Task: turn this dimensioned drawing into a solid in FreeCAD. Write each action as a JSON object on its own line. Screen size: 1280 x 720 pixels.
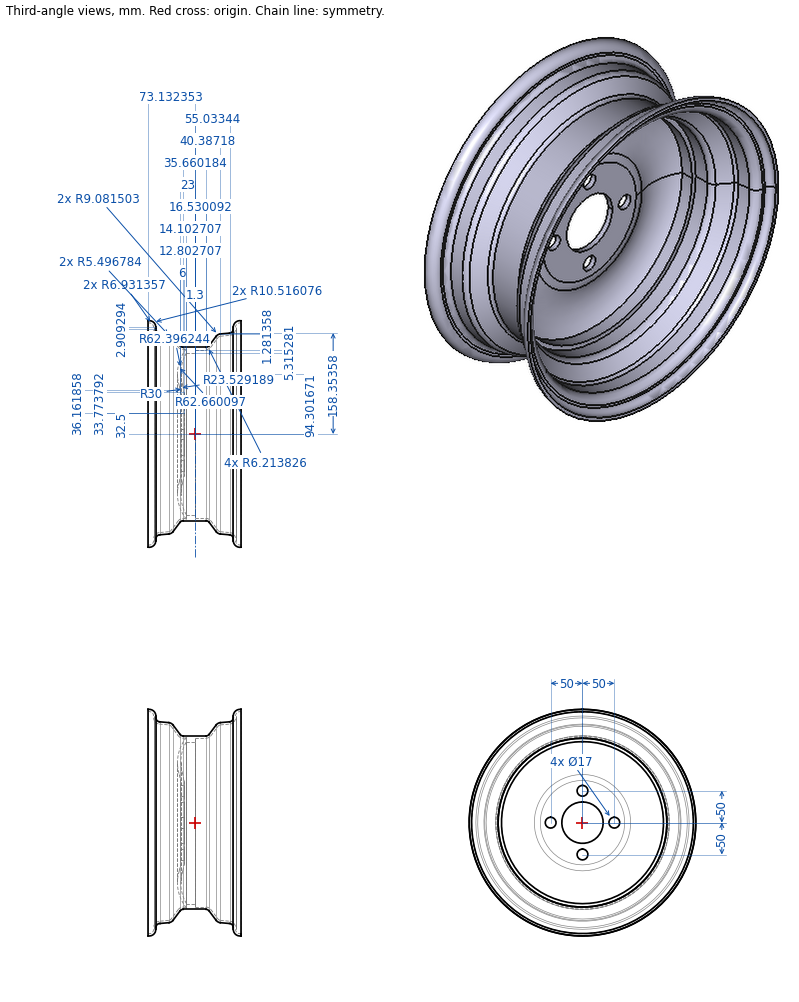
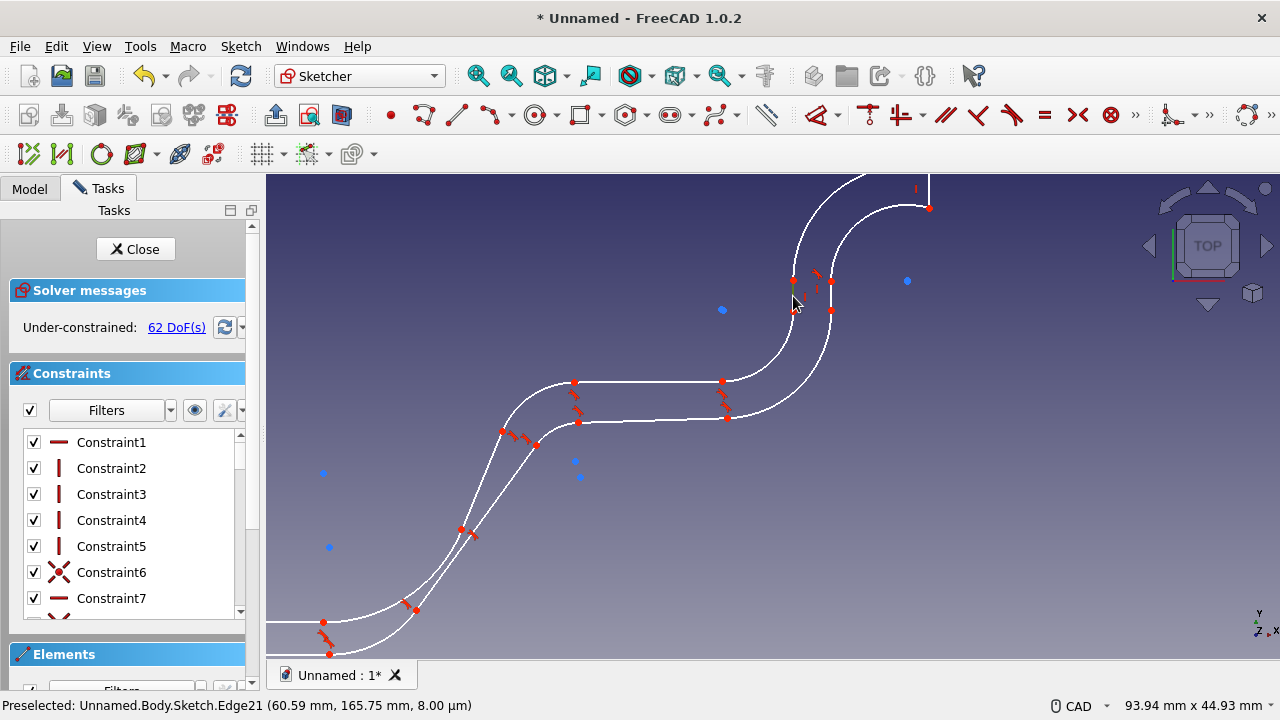
{"action": "left_click", "coordinate": [809, 223]}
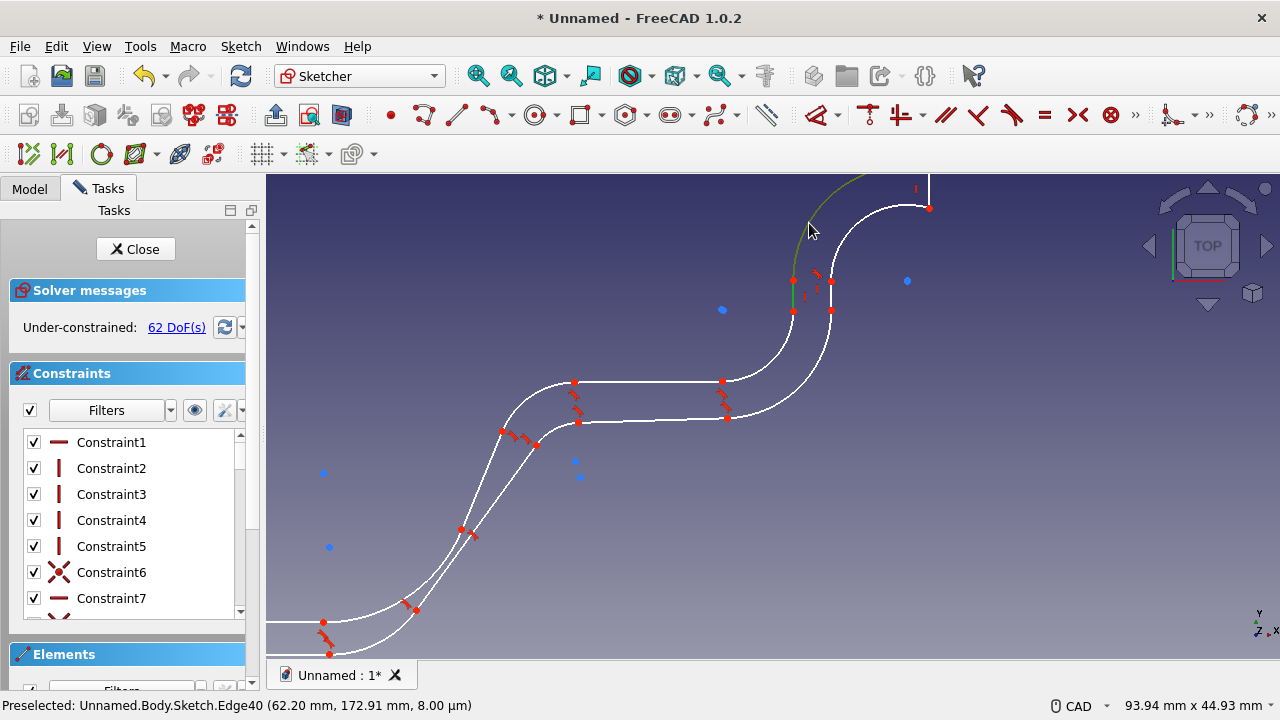
{"action": "key", "text": "t"}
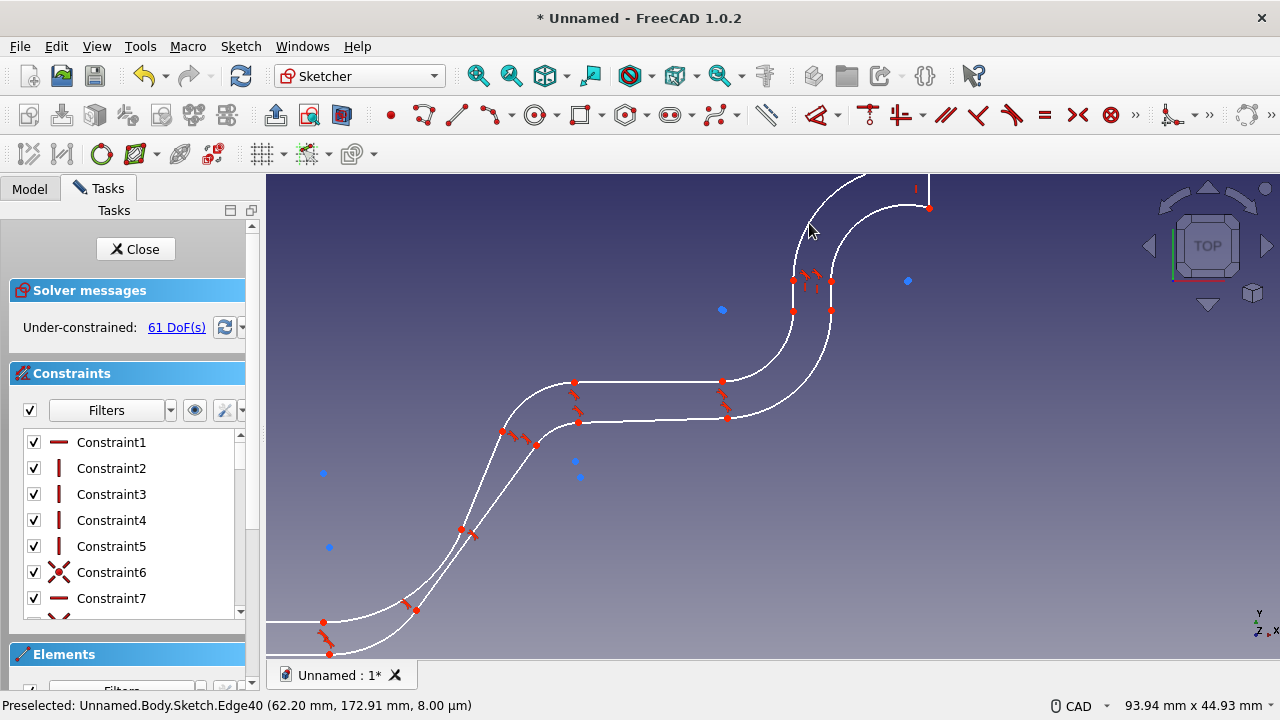
{"action": "scroll", "coordinate": [793, 290], "scroll_direction": "up", "scroll_amount": 2}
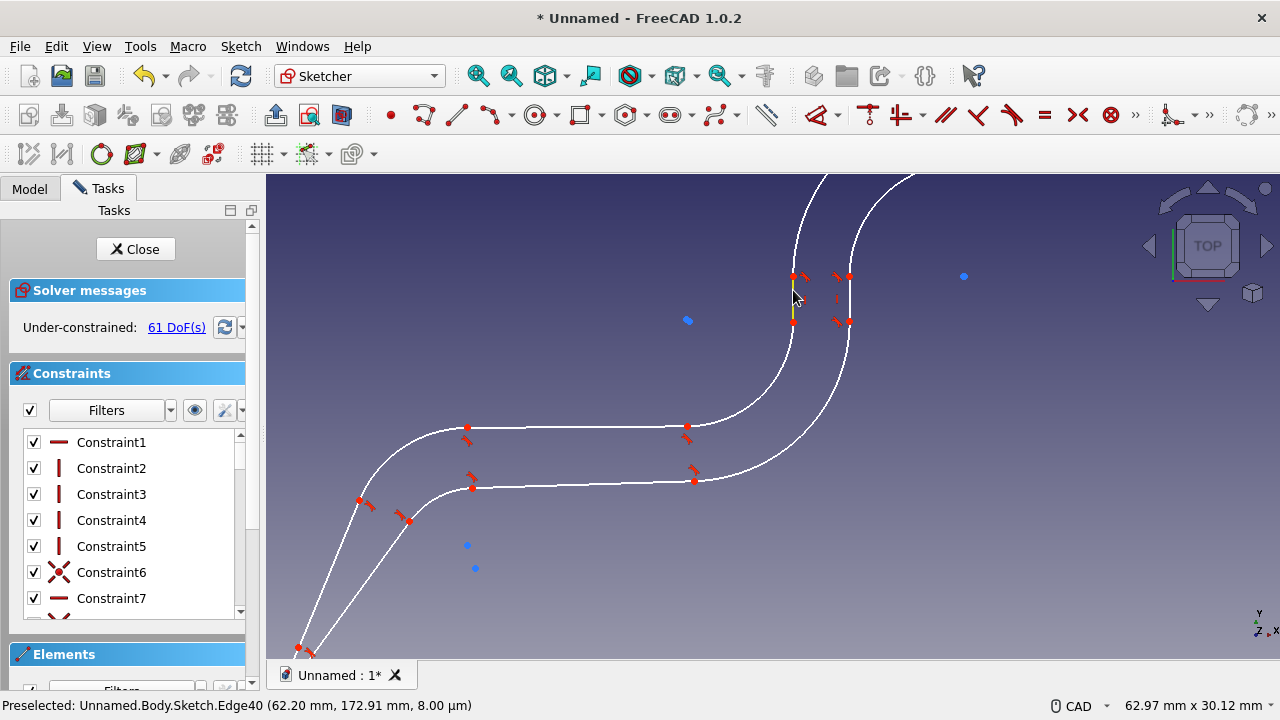
{"action": "left_click", "coordinate": [793, 290]}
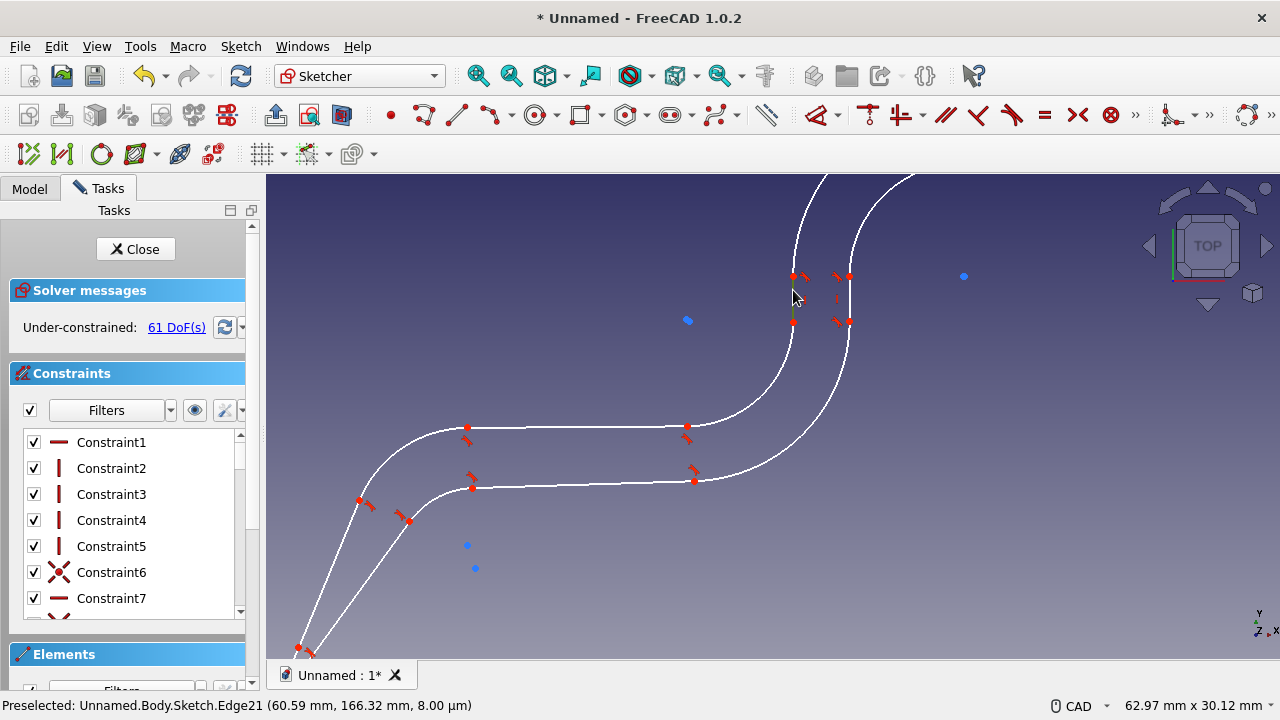
{"action": "scroll", "coordinate": [815, 277], "scroll_direction": "down", "scroll_amount": 11}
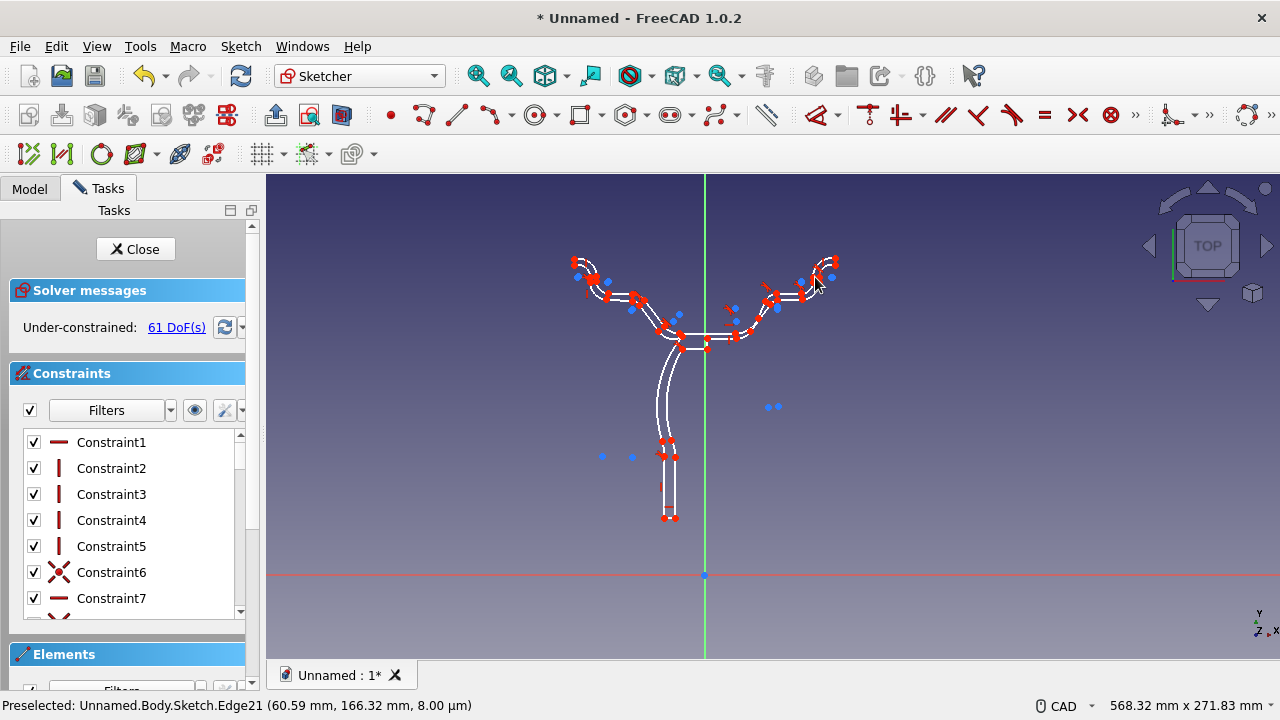
{"action": "scroll", "coordinate": [807, 292], "scroll_direction": "up", "scroll_amount": 5}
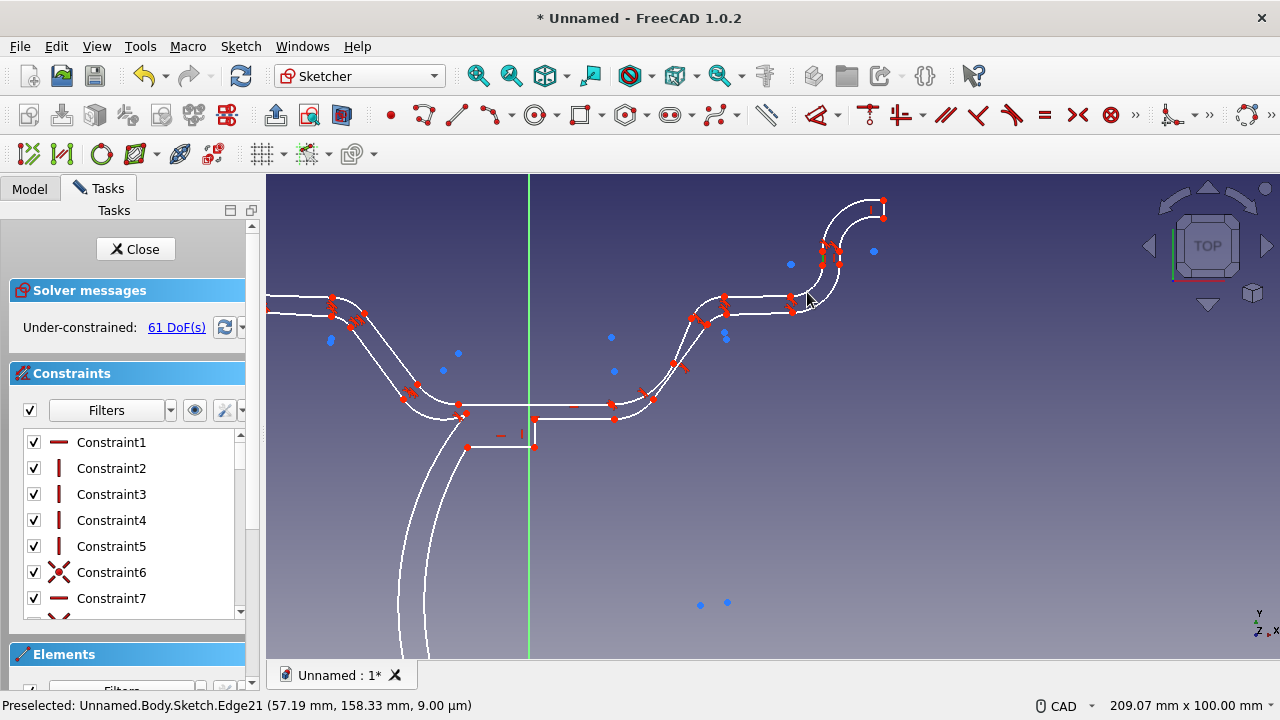
{"action": "left_click", "coordinate": [805, 293]}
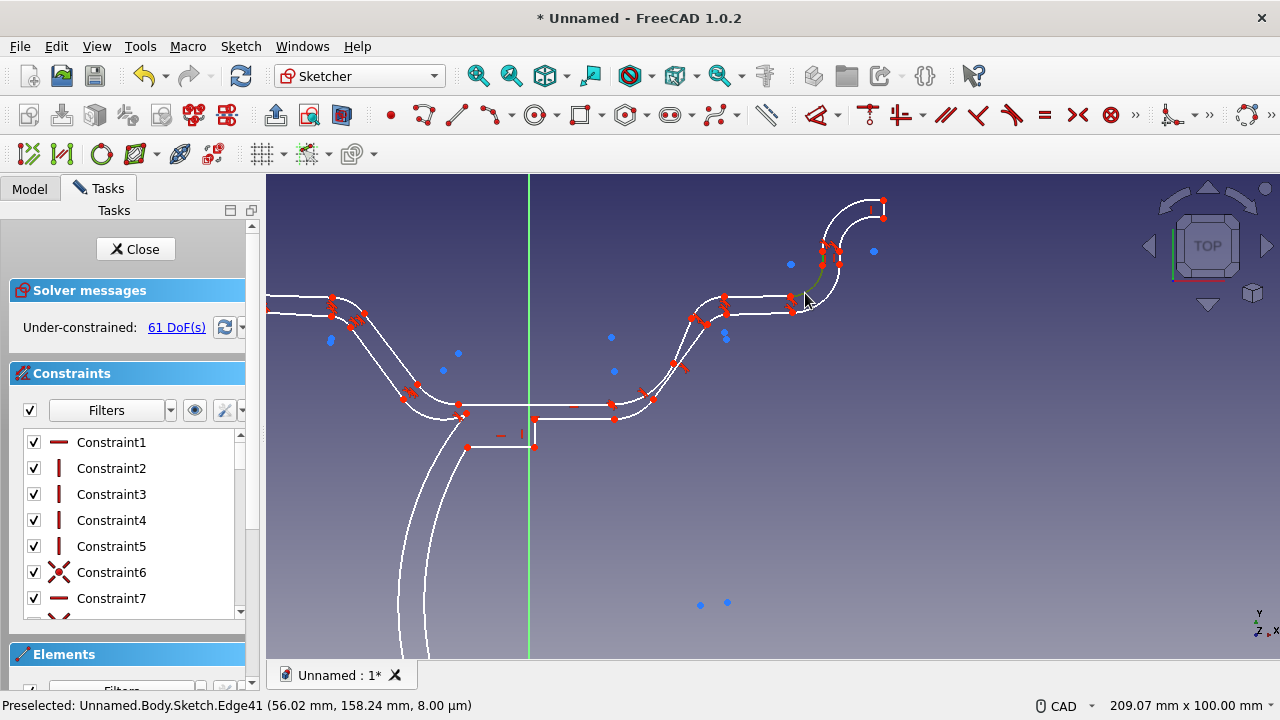
{"action": "key", "text": "t"}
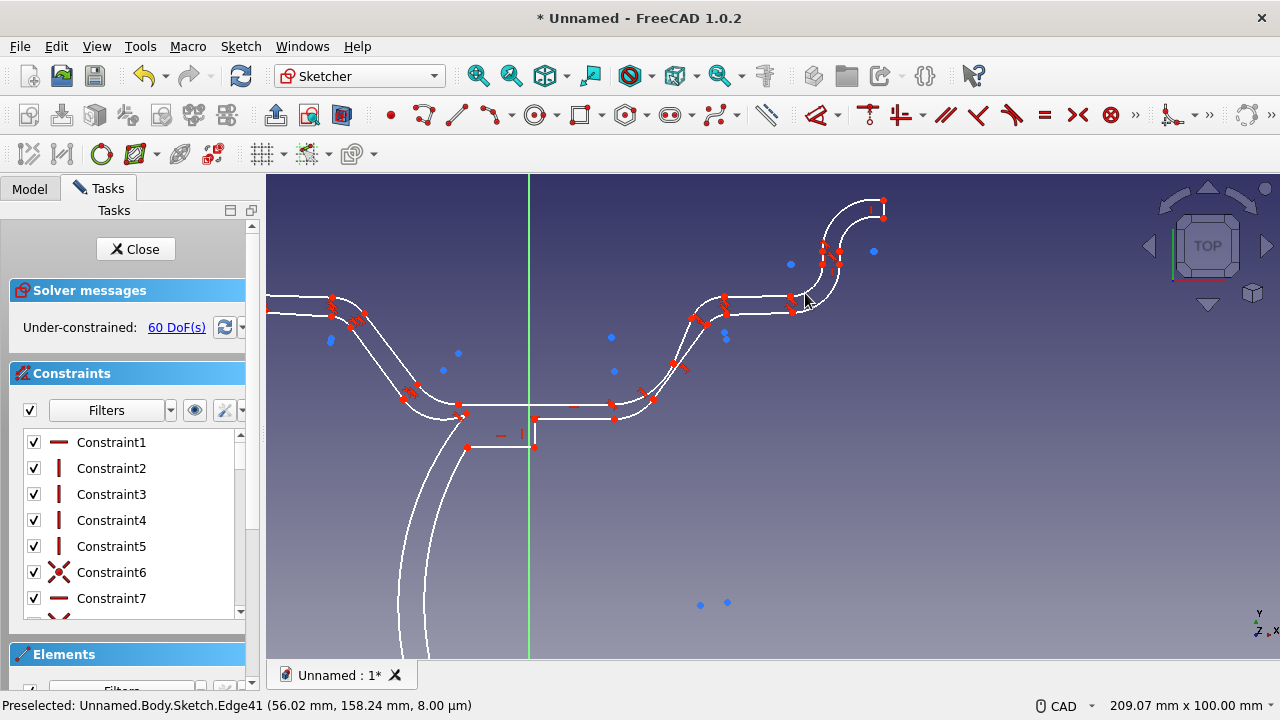
{"action": "left_click", "coordinate": [421, 491]}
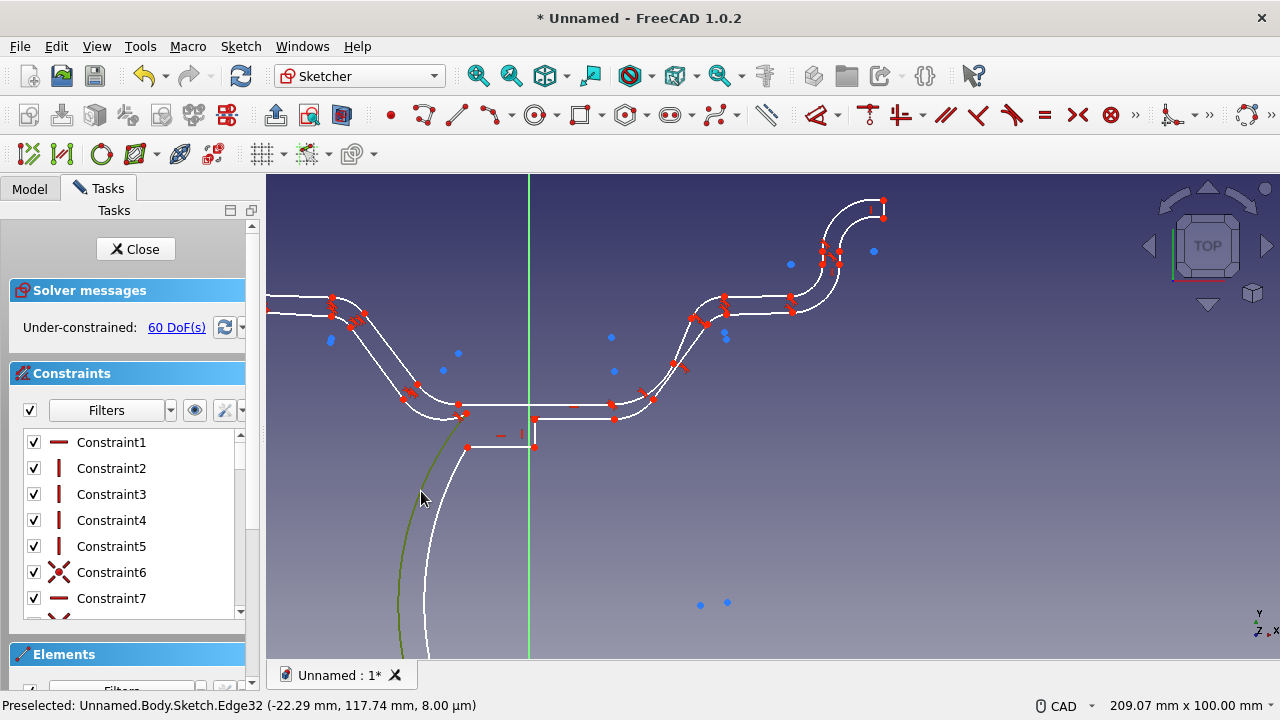
{"action": "scroll", "coordinate": [807, 292], "scroll_direction": "down", "scroll_amount": 5}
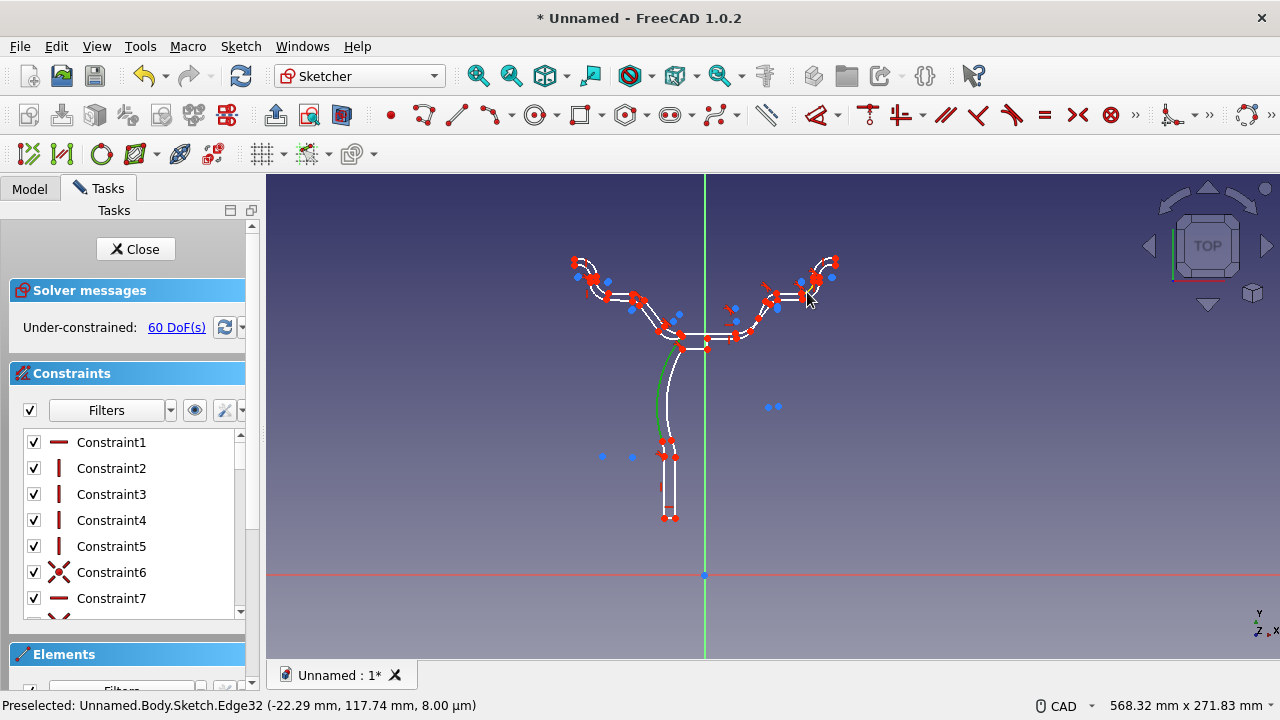
{"action": "scroll", "coordinate": [664, 452], "scroll_direction": "up", "scroll_amount": 6}